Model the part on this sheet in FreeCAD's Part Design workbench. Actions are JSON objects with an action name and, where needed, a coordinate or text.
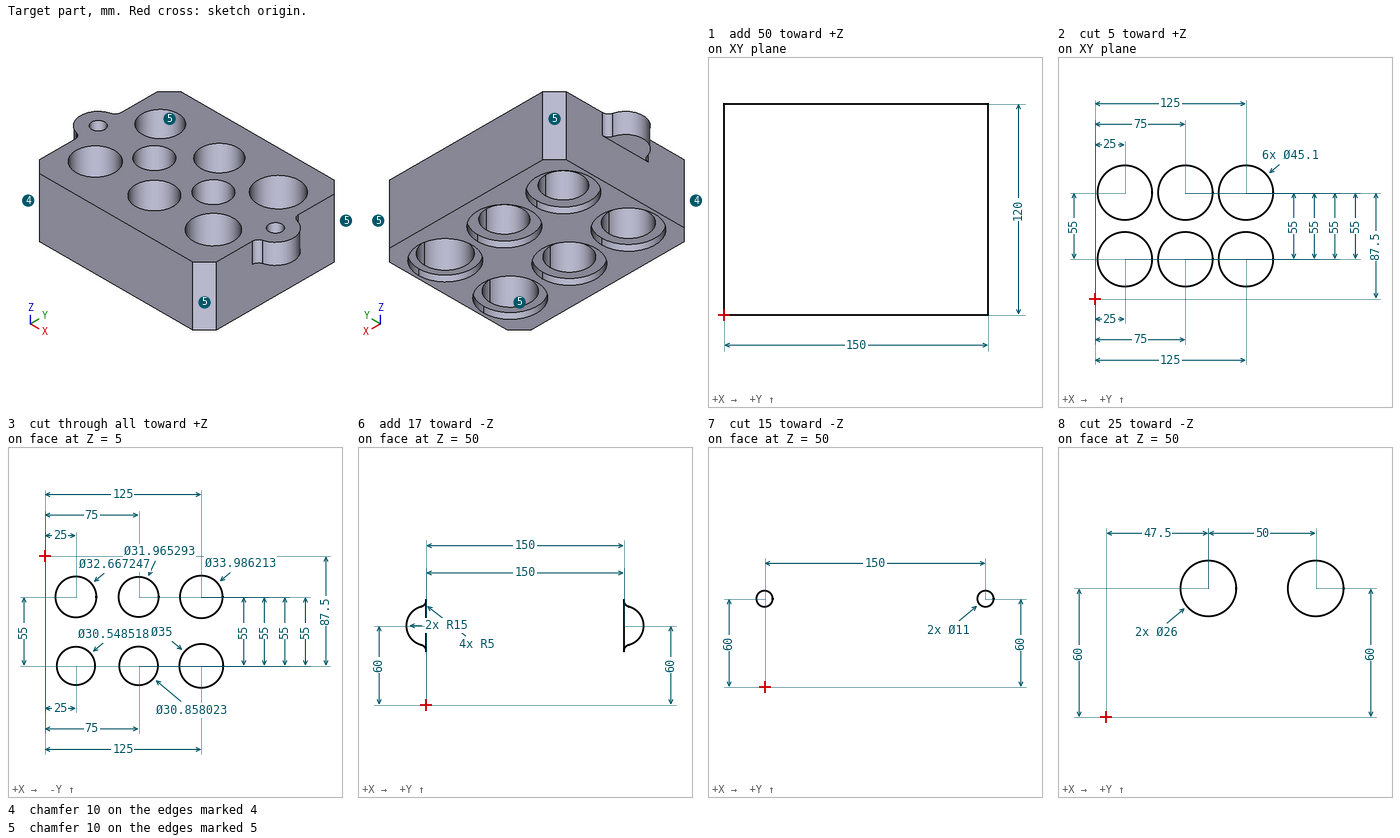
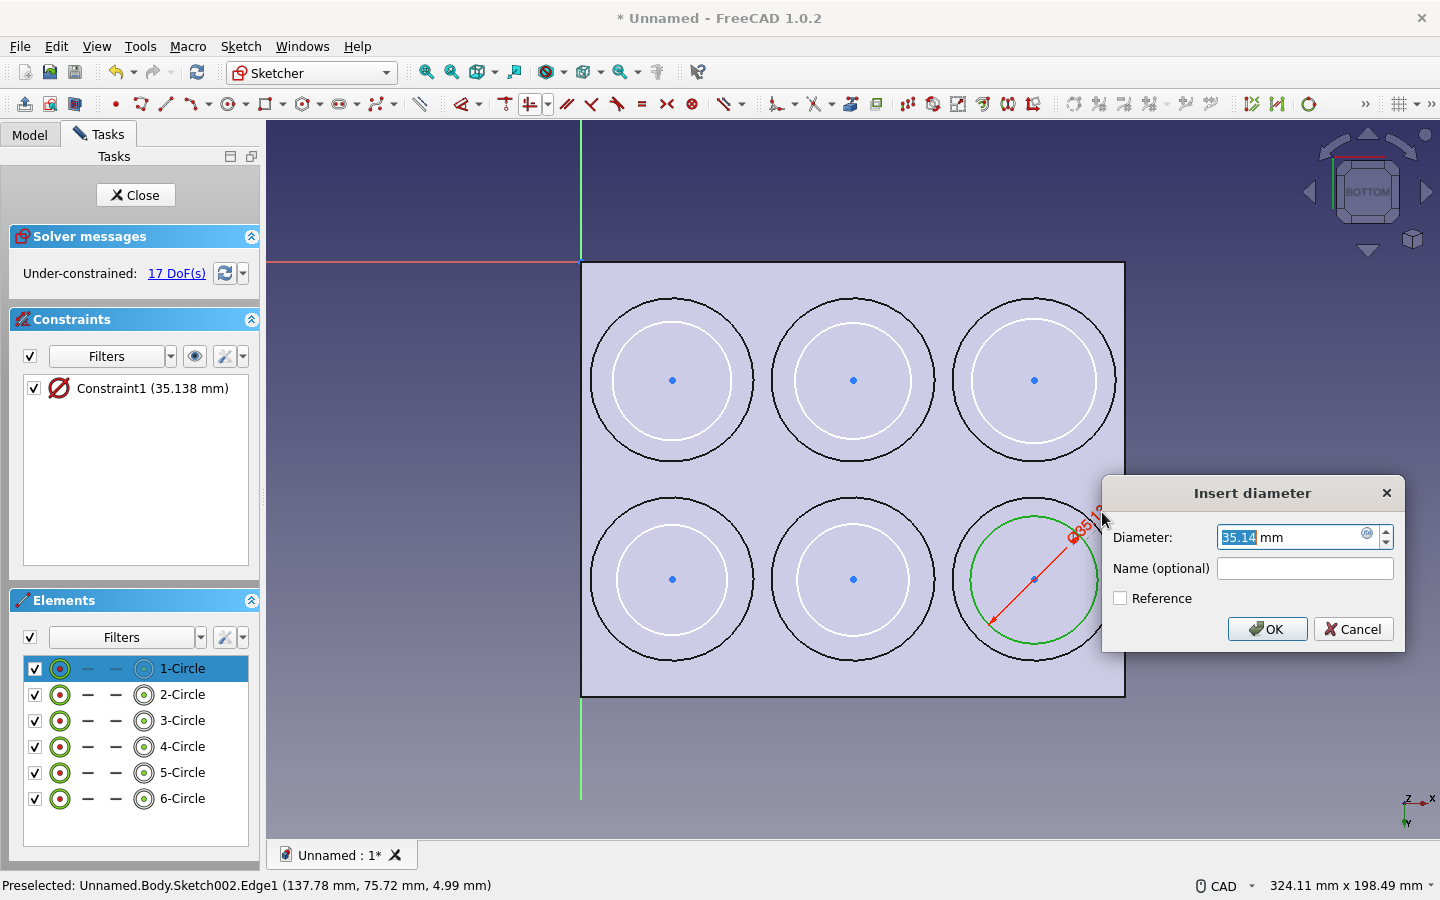
{"action": "type", "text": "35"}
{"action": "key", "text": "Return"}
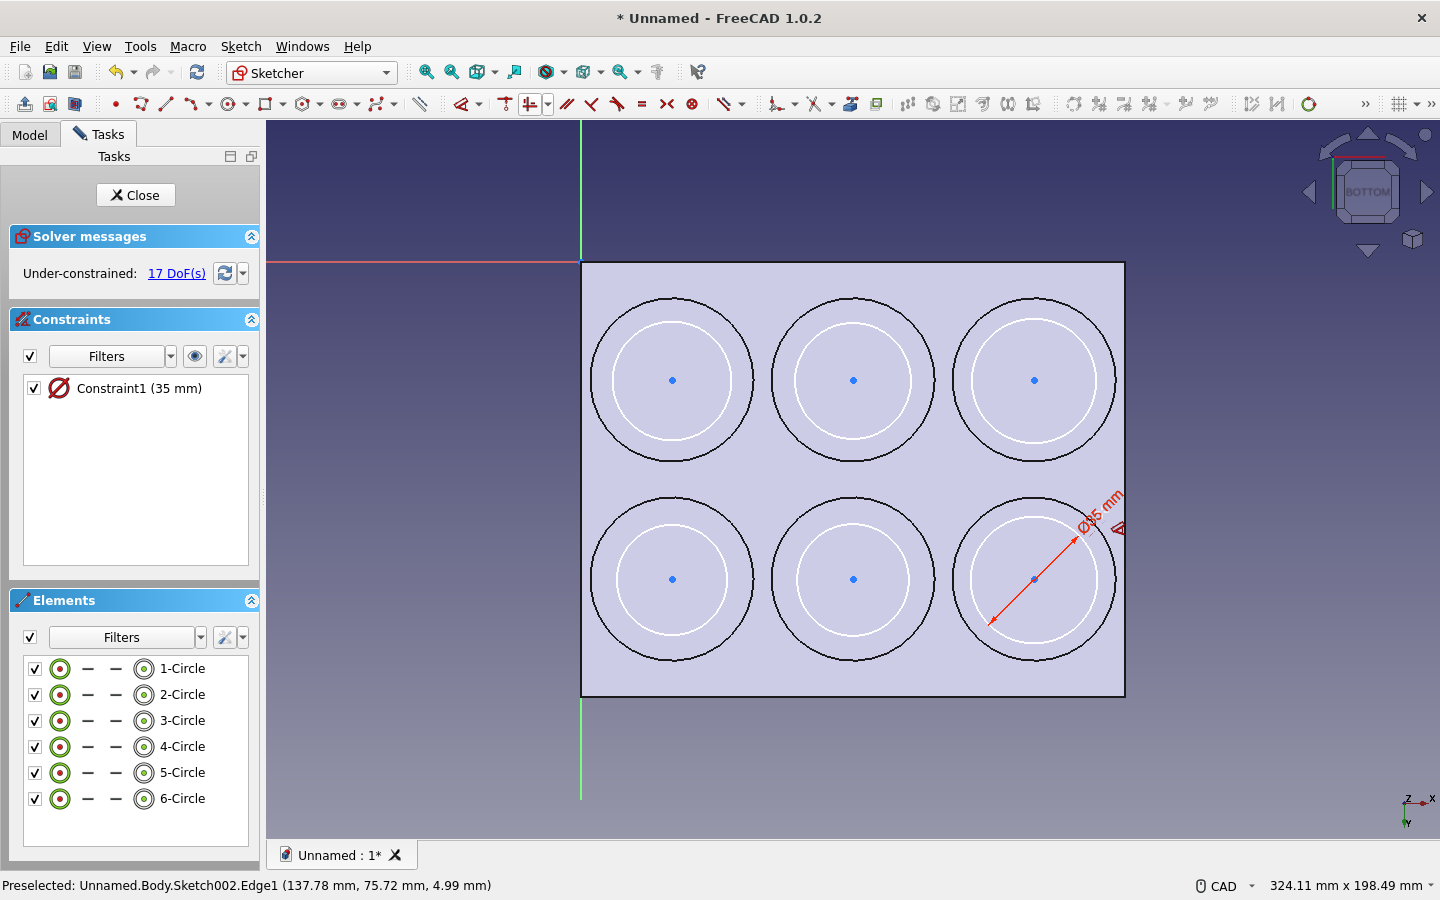
{"action": "left_click", "coordinate": [892, 540]}
{"action": "left_click", "coordinate": [914, 517]}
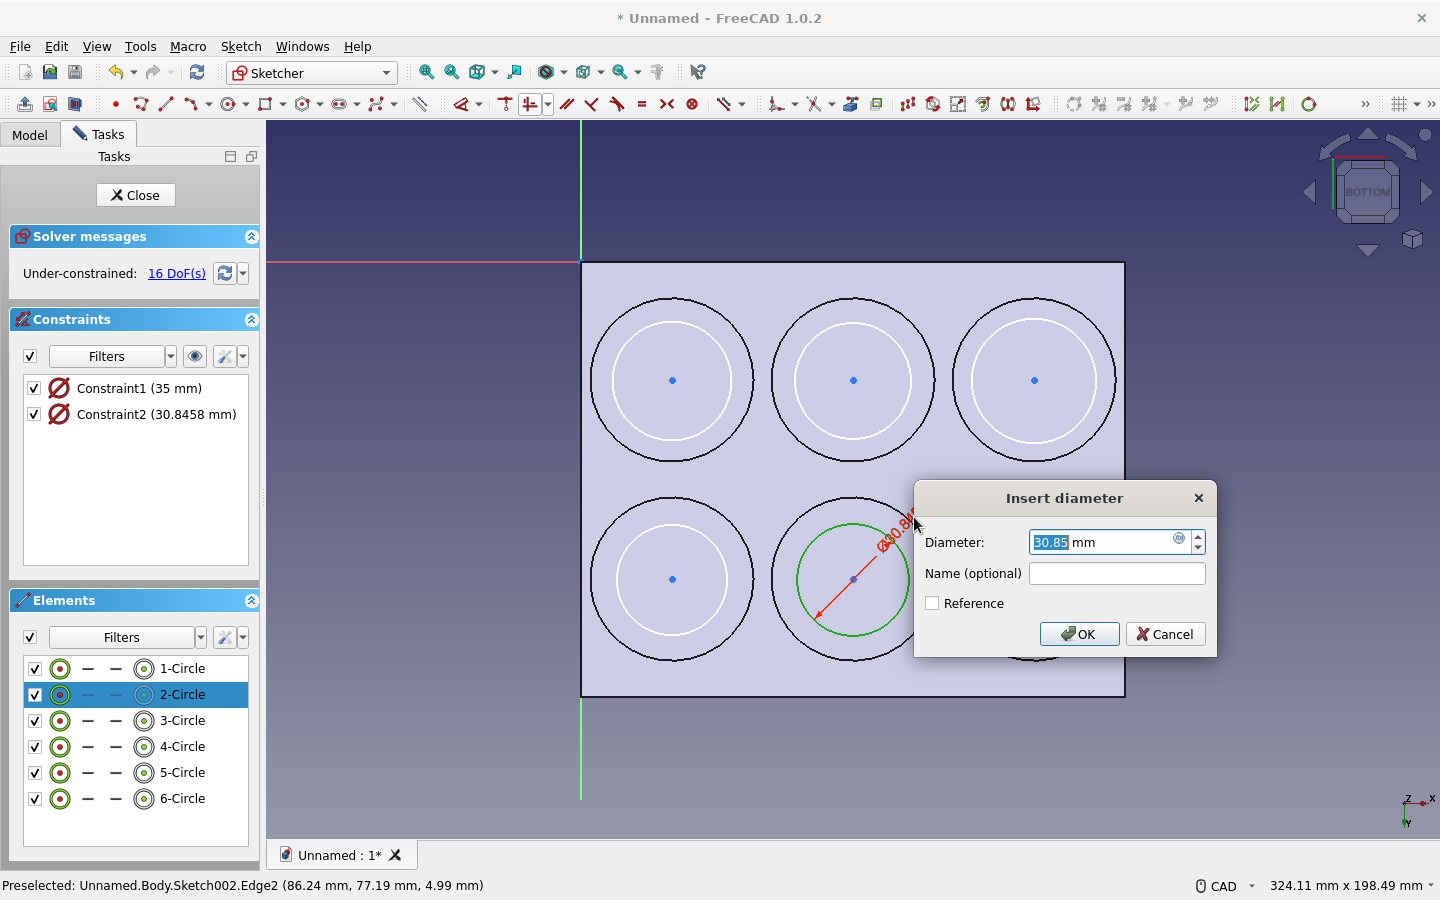
{"action": "type", "text": "30.858023"}
{"action": "key", "text": "Return"}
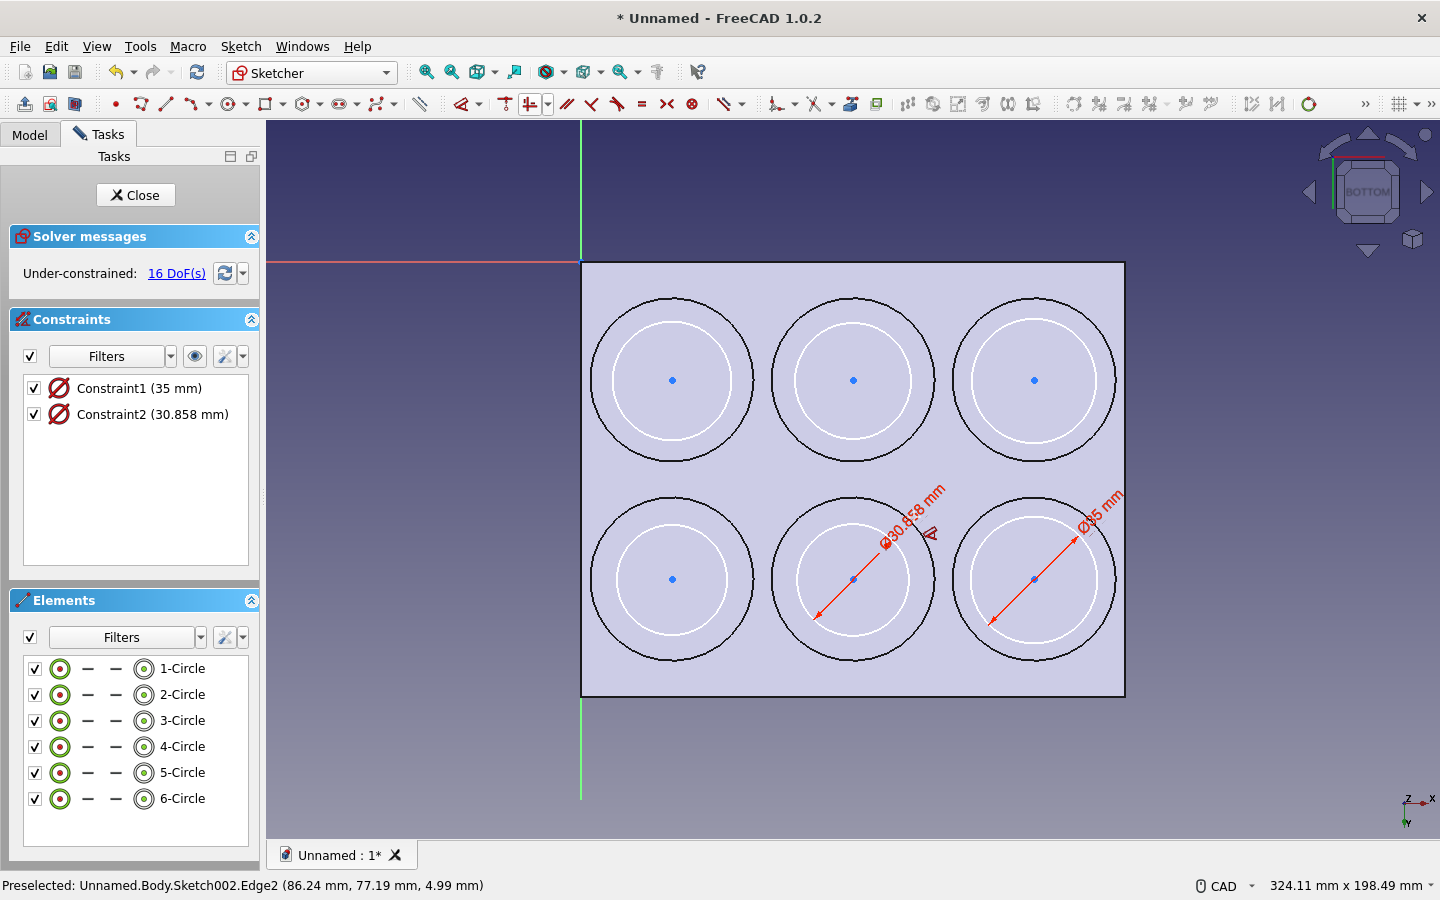
{"action": "left_click", "coordinate": [711, 541]}
{"action": "left_click", "coordinate": [734, 518]}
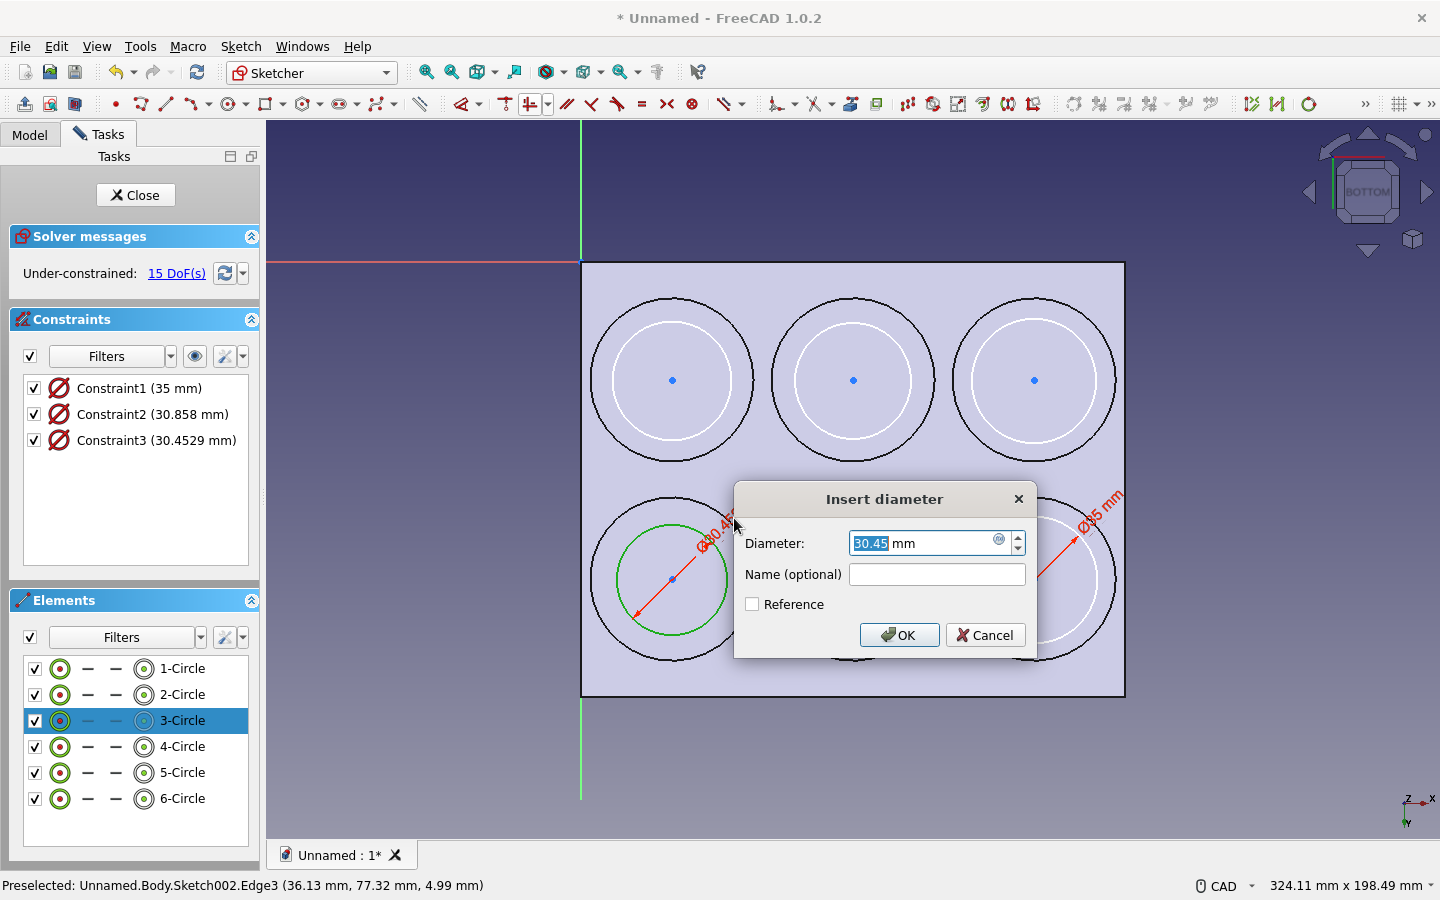
{"action": "type", "text": "30.548518"}
{"action": "key", "text": "Return"}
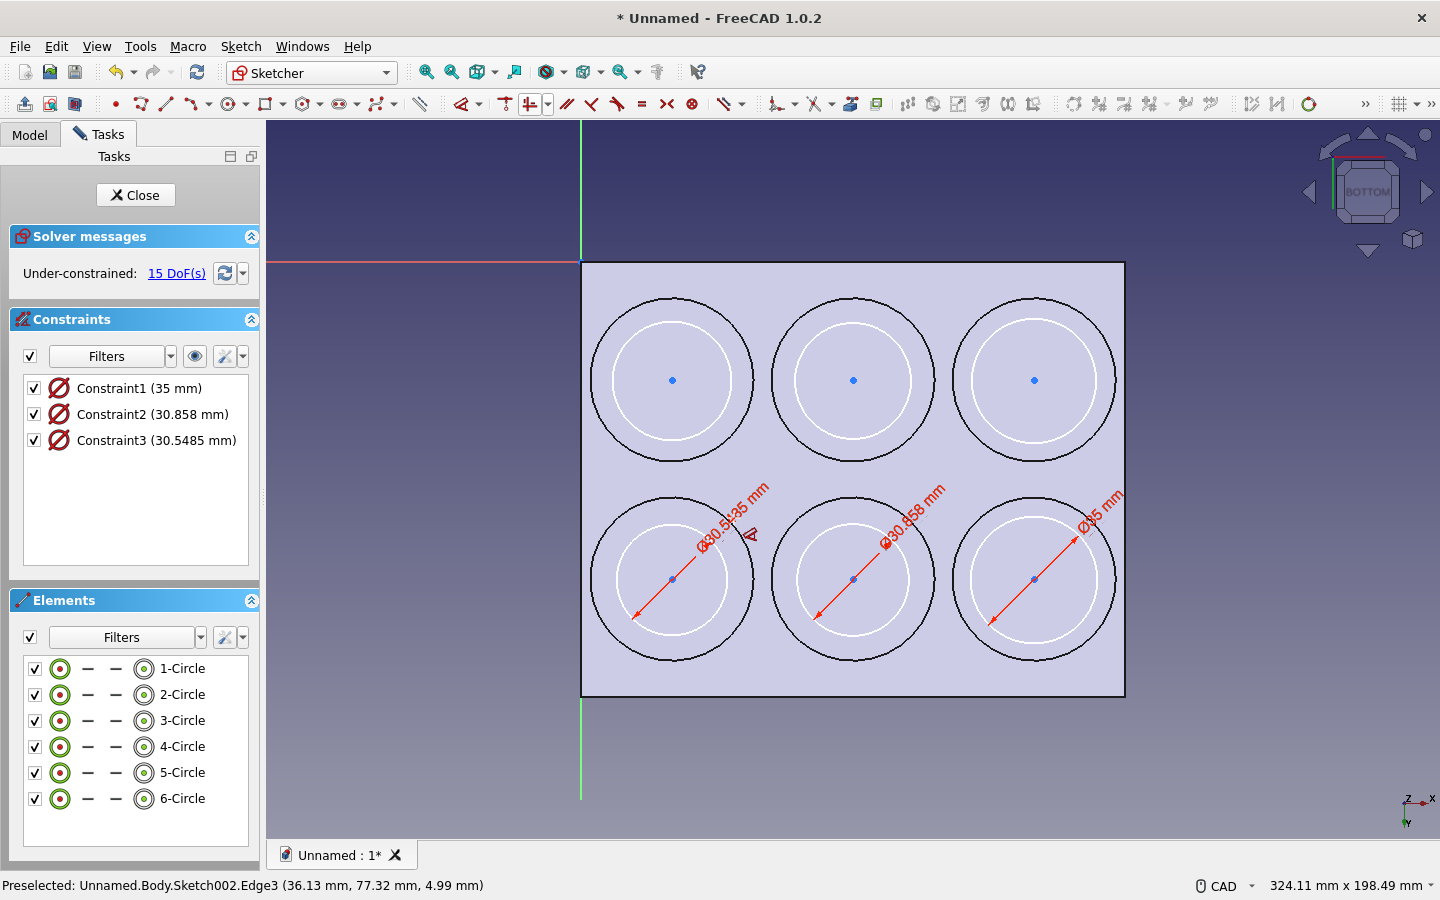
{"action": "left_click", "coordinate": [1078, 337]}
{"action": "left_click", "coordinate": [1101, 314]}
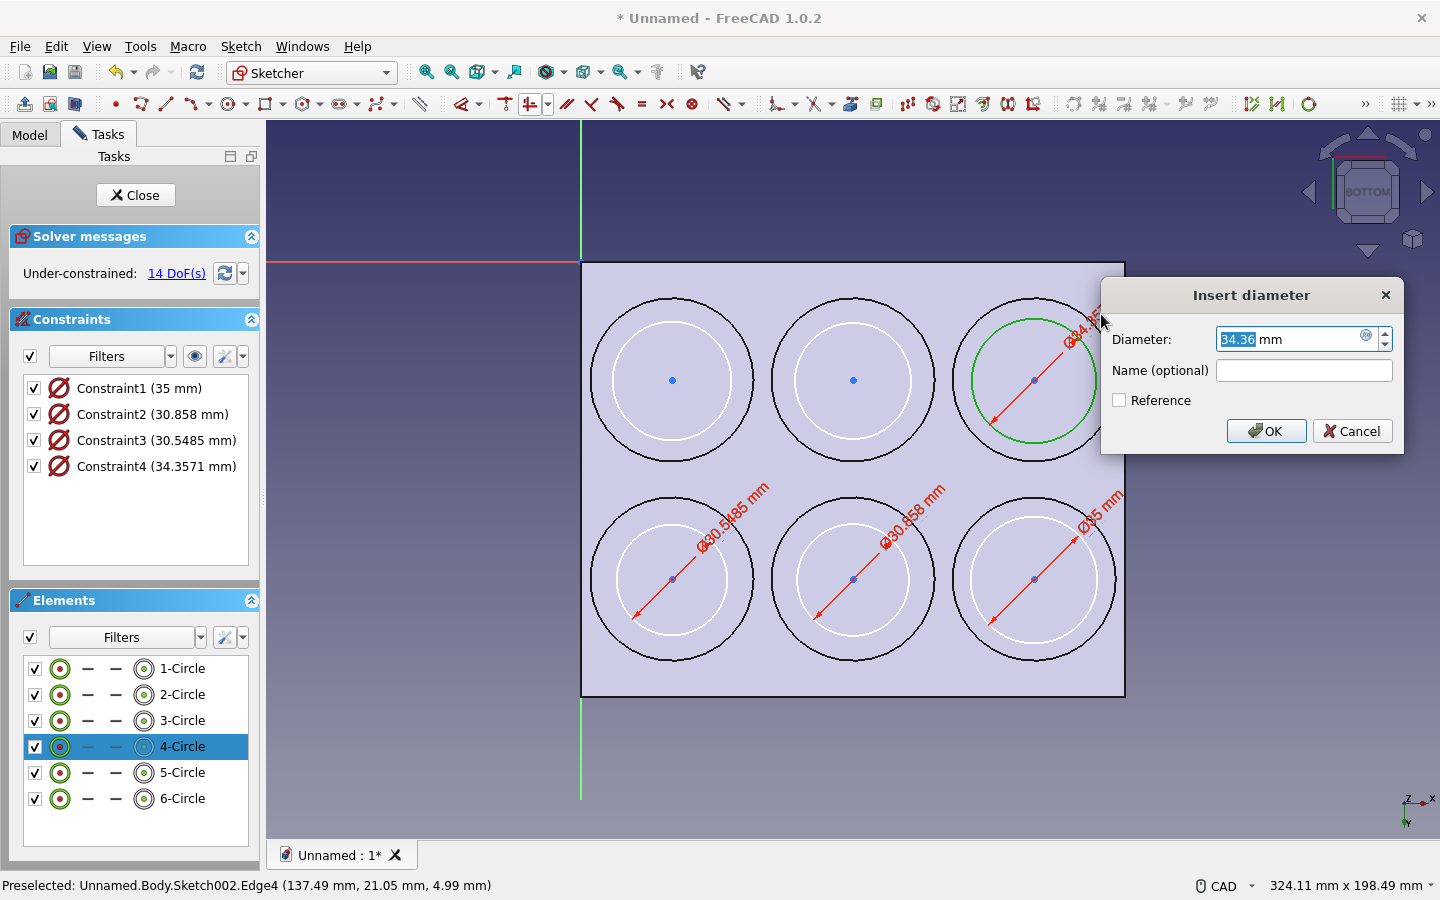
{"action": "type", "text": "33.986213"}
{"action": "key", "text": "Return"}